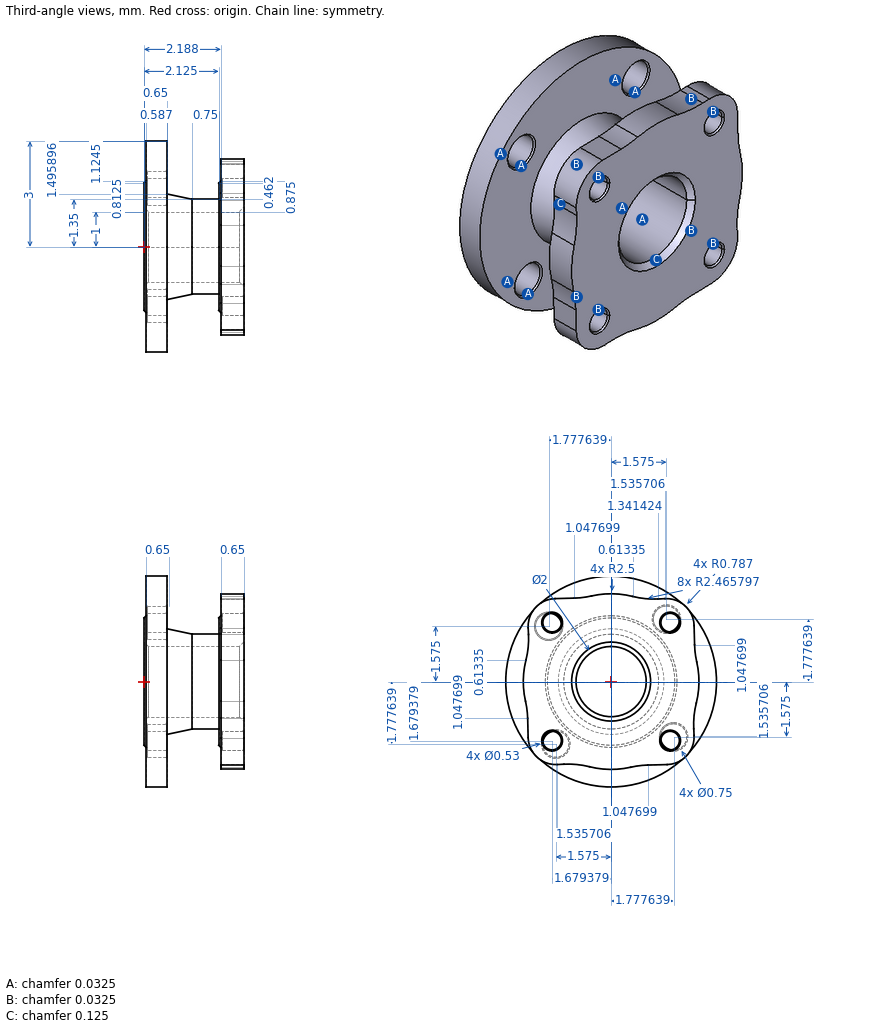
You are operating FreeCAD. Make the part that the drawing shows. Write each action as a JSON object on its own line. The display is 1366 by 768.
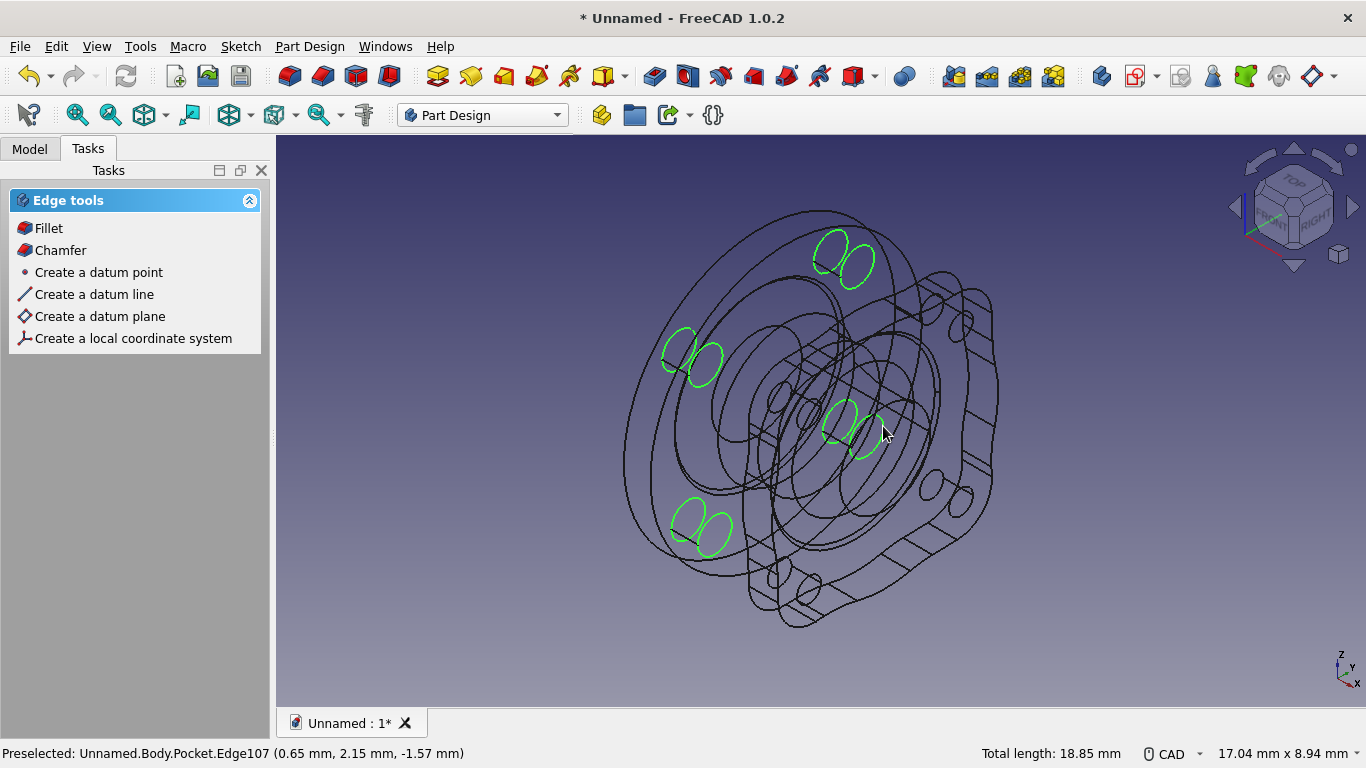
{"action": "key", "text": "v 1"}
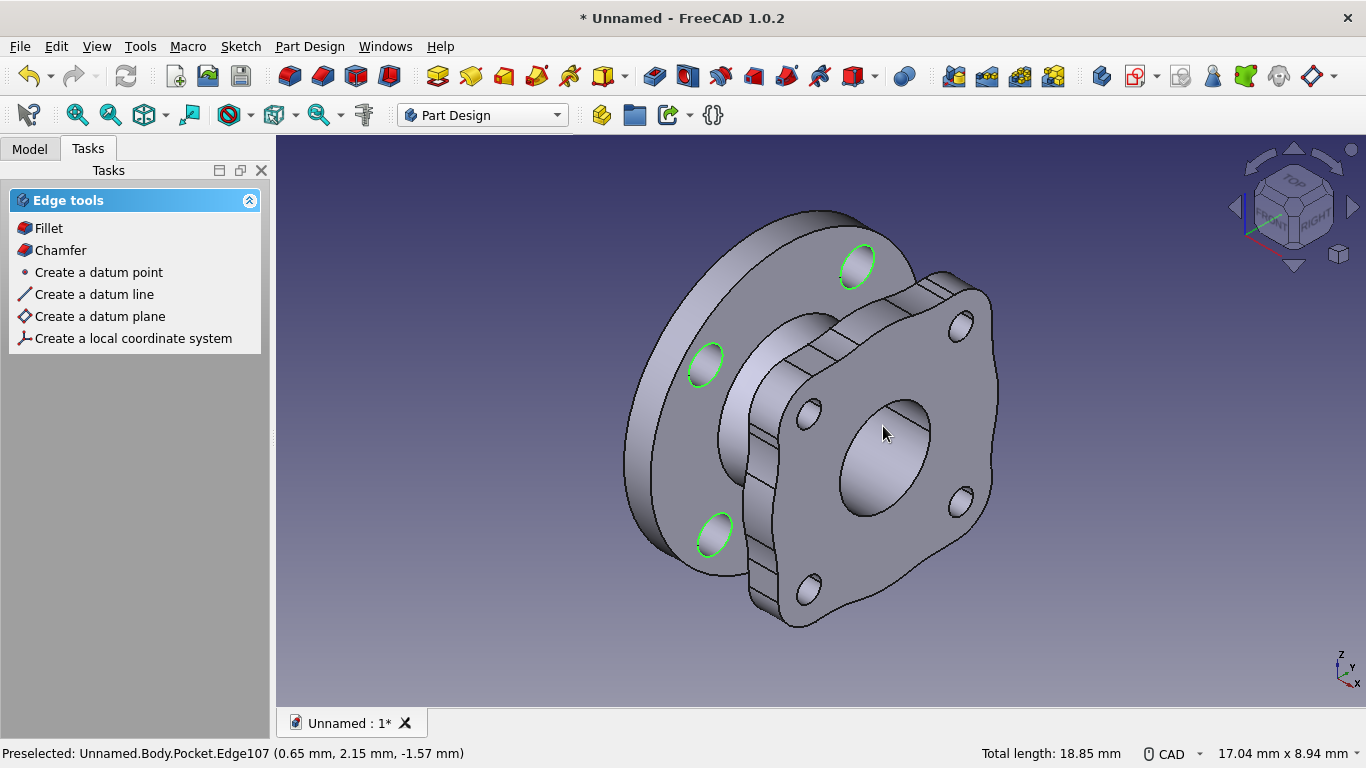
{"action": "left_click", "coordinate": [323, 76]}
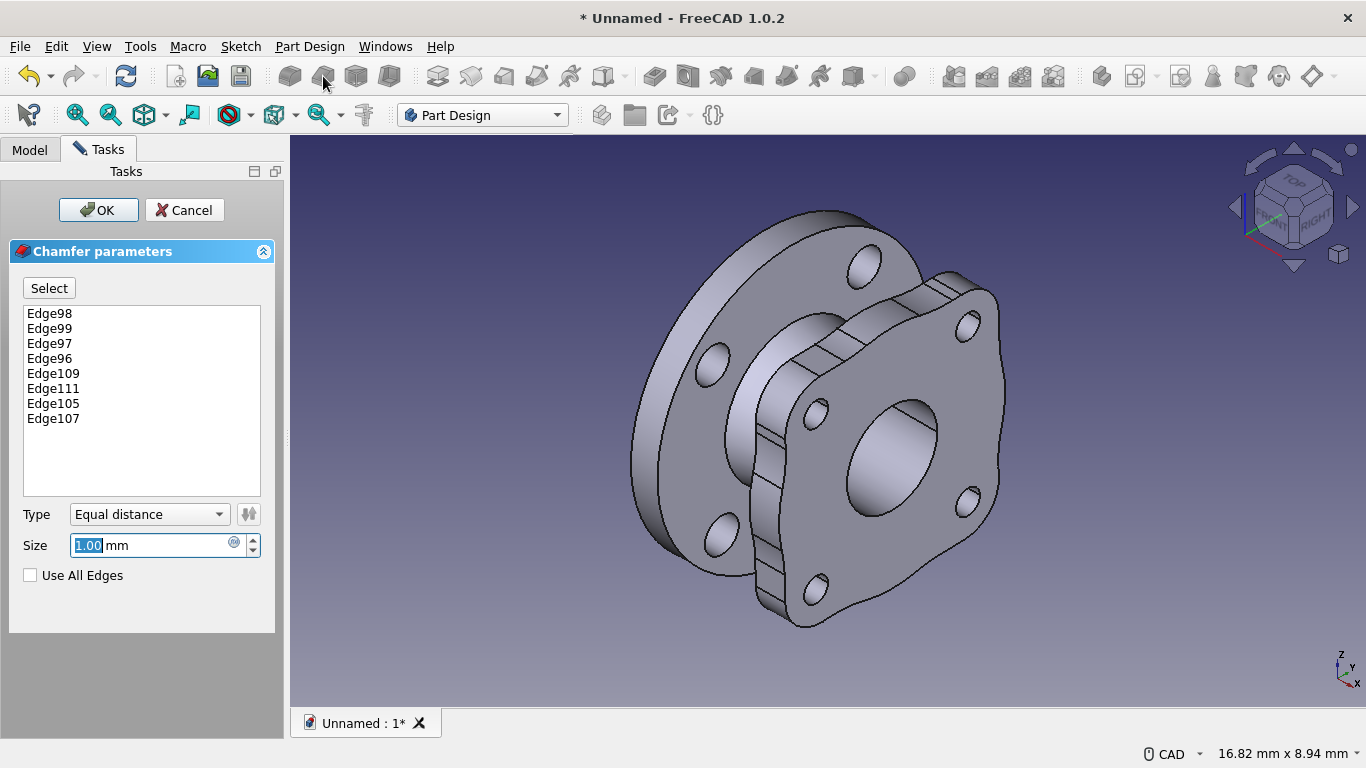
{"action": "type", "text": "0.0325"}
{"action": "key", "text": "Tab"}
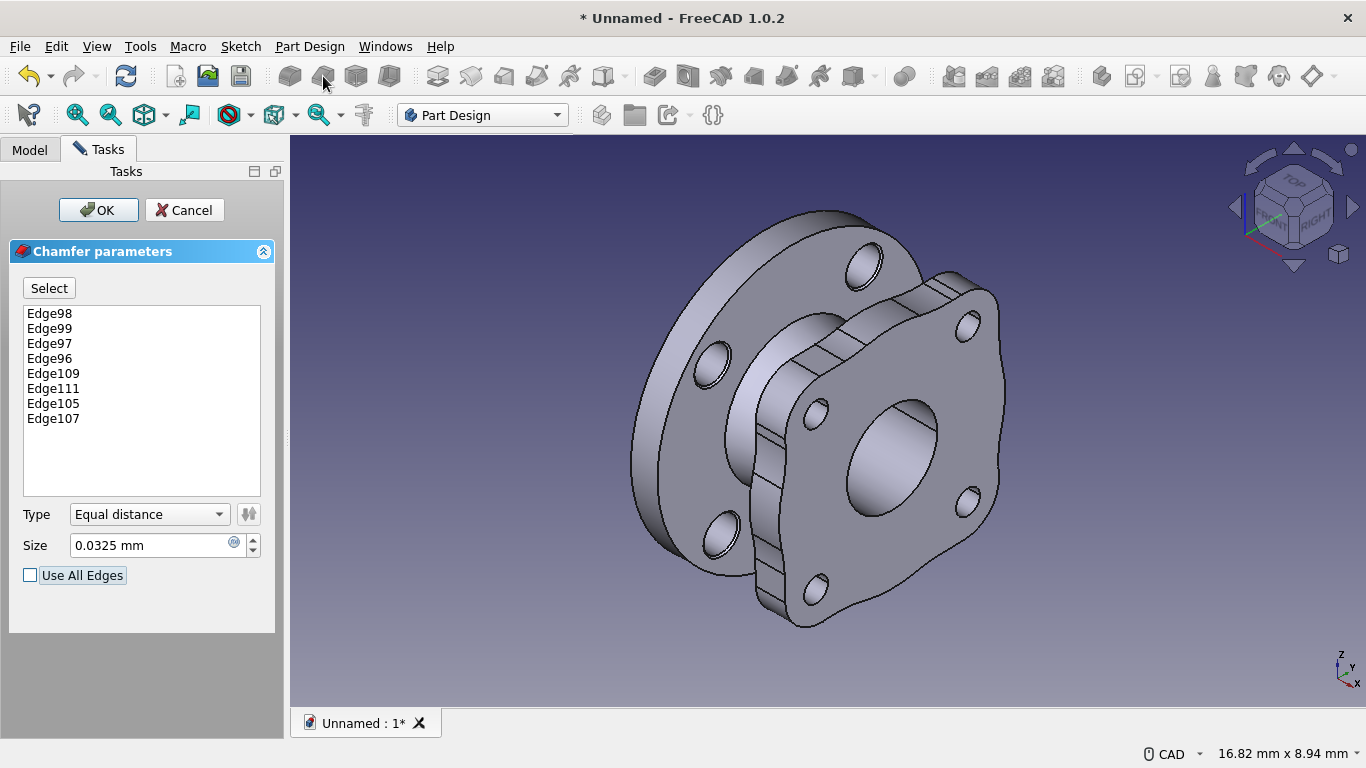
{"action": "left_click", "coordinate": [99, 210]}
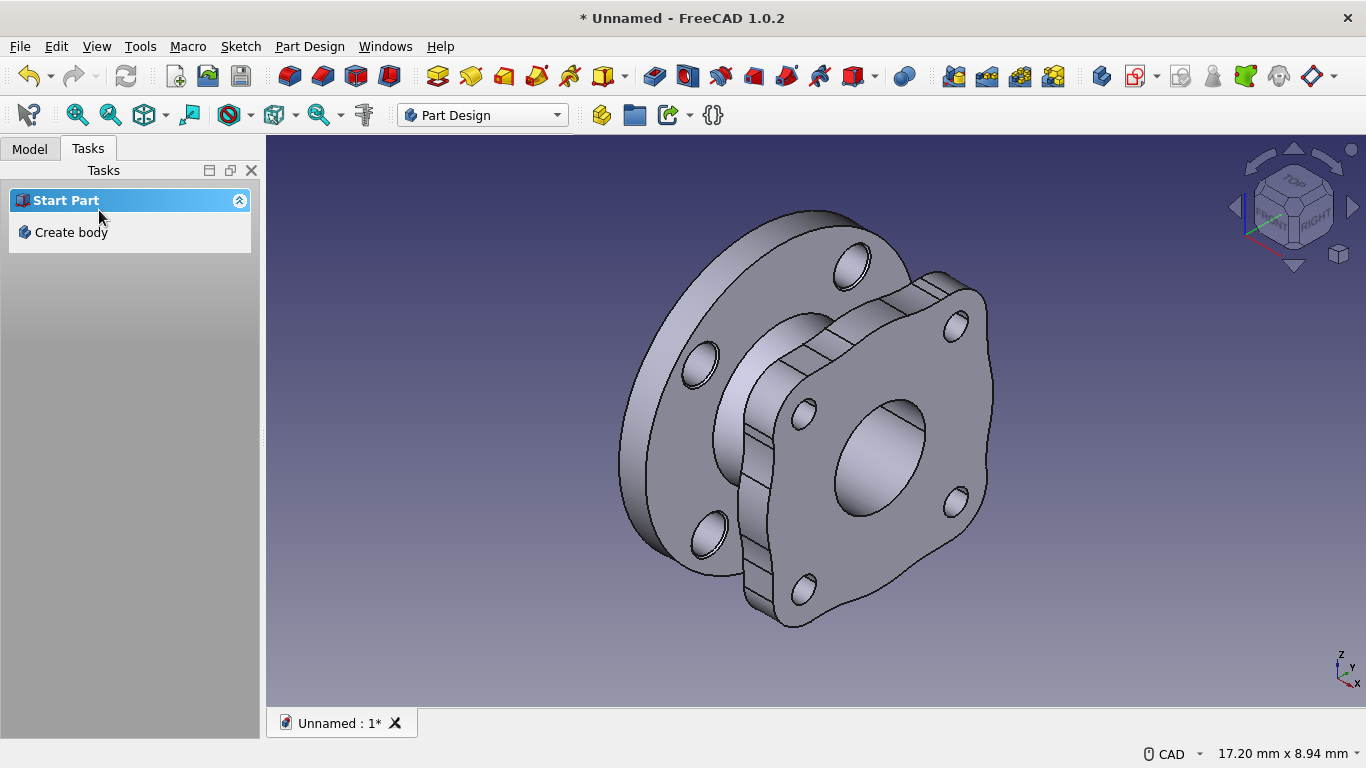
{"action": "left_click", "coordinate": [946, 339]}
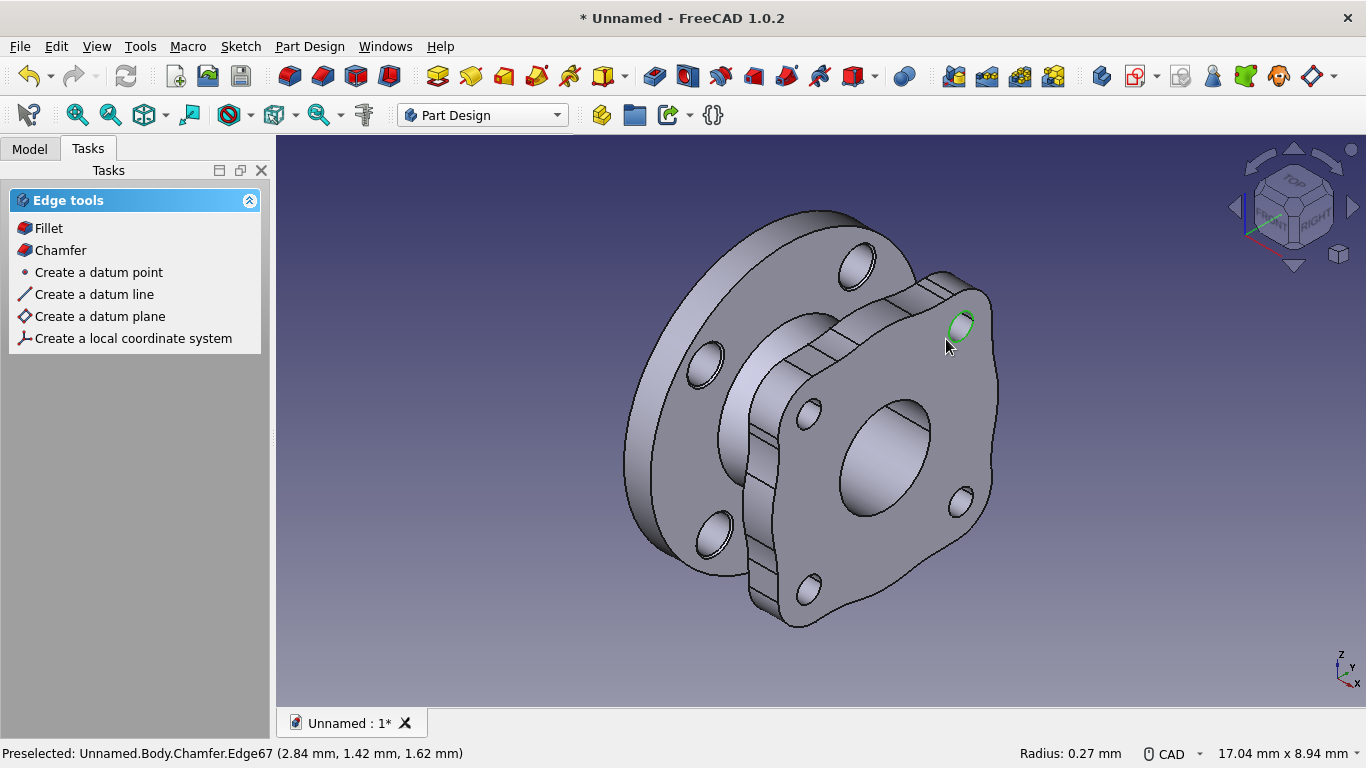
{"action": "left_click", "coordinate": [951, 515], "text": "ctrl"}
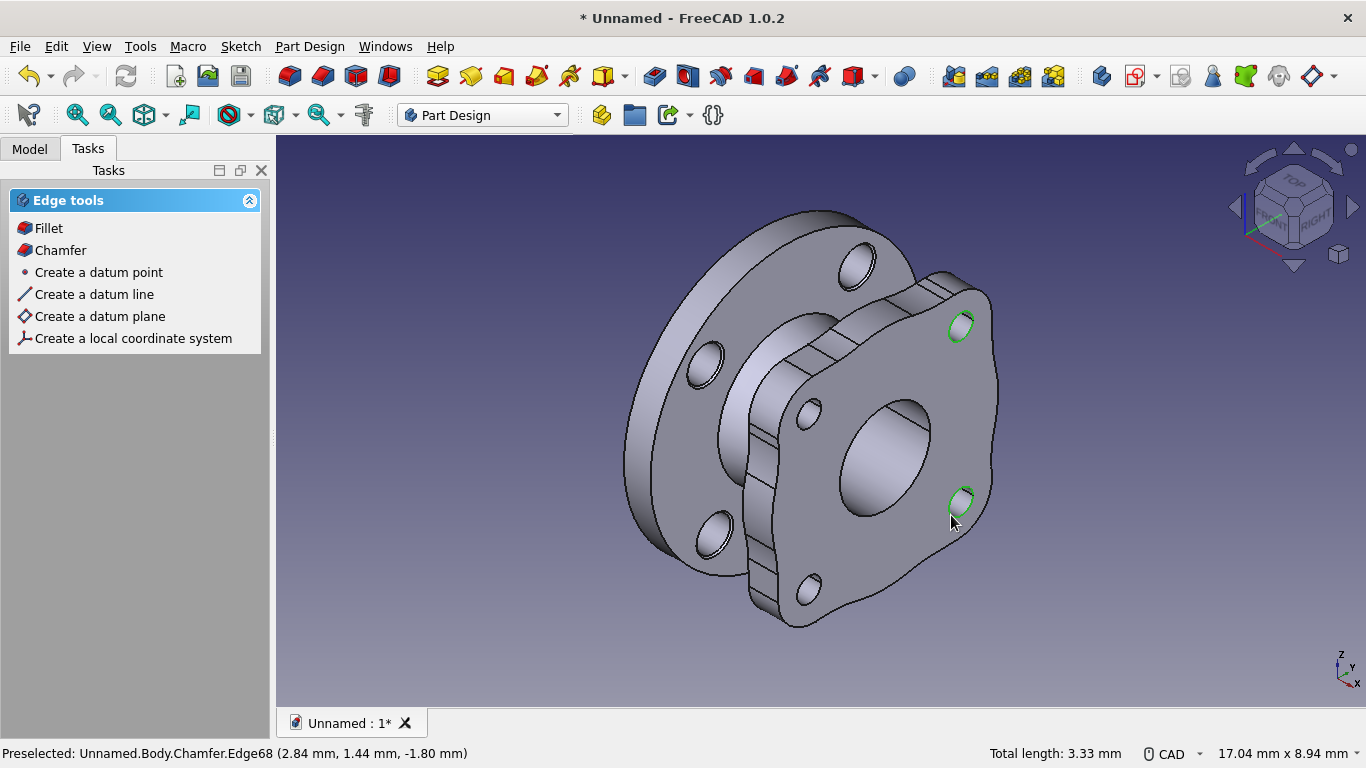
{"action": "left_click", "coordinate": [799, 602], "text": "ctrl"}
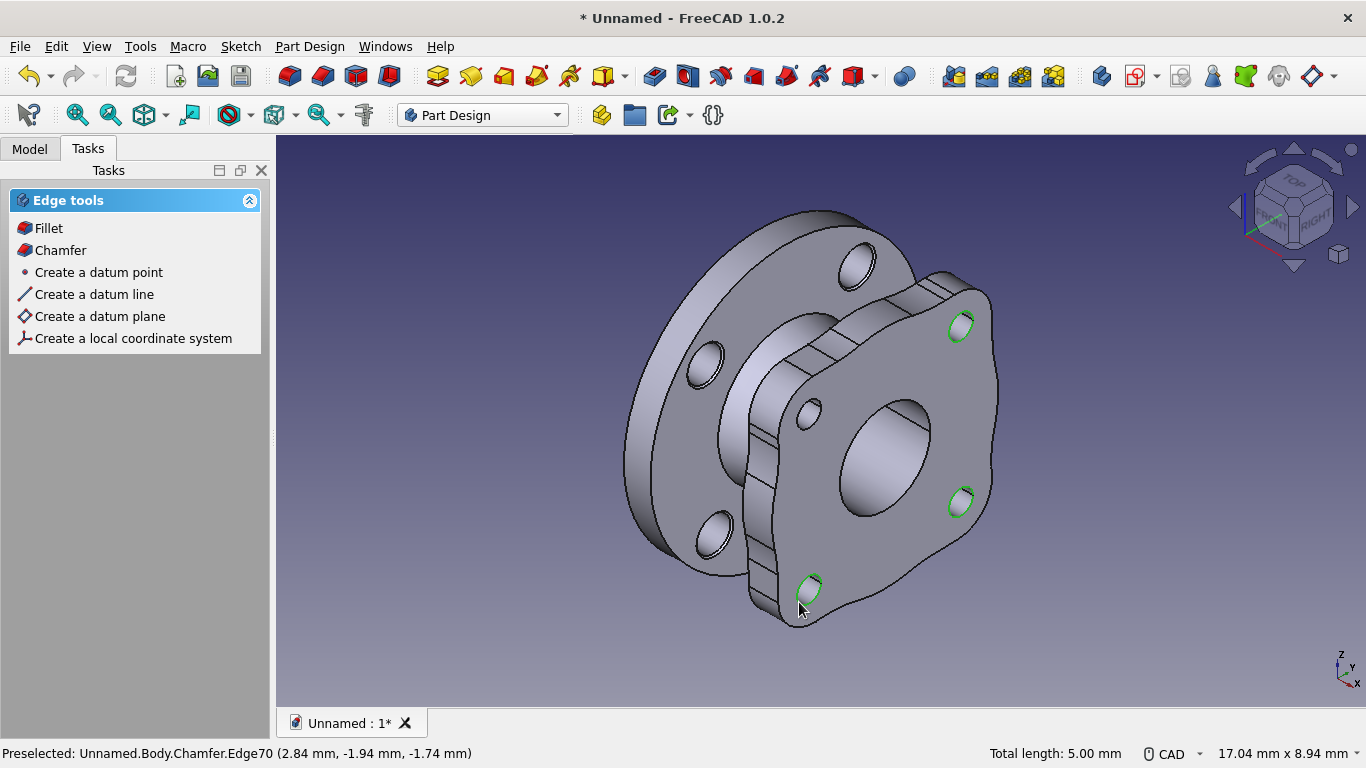
{"action": "left_click", "coordinate": [799, 427], "text": "ctrl"}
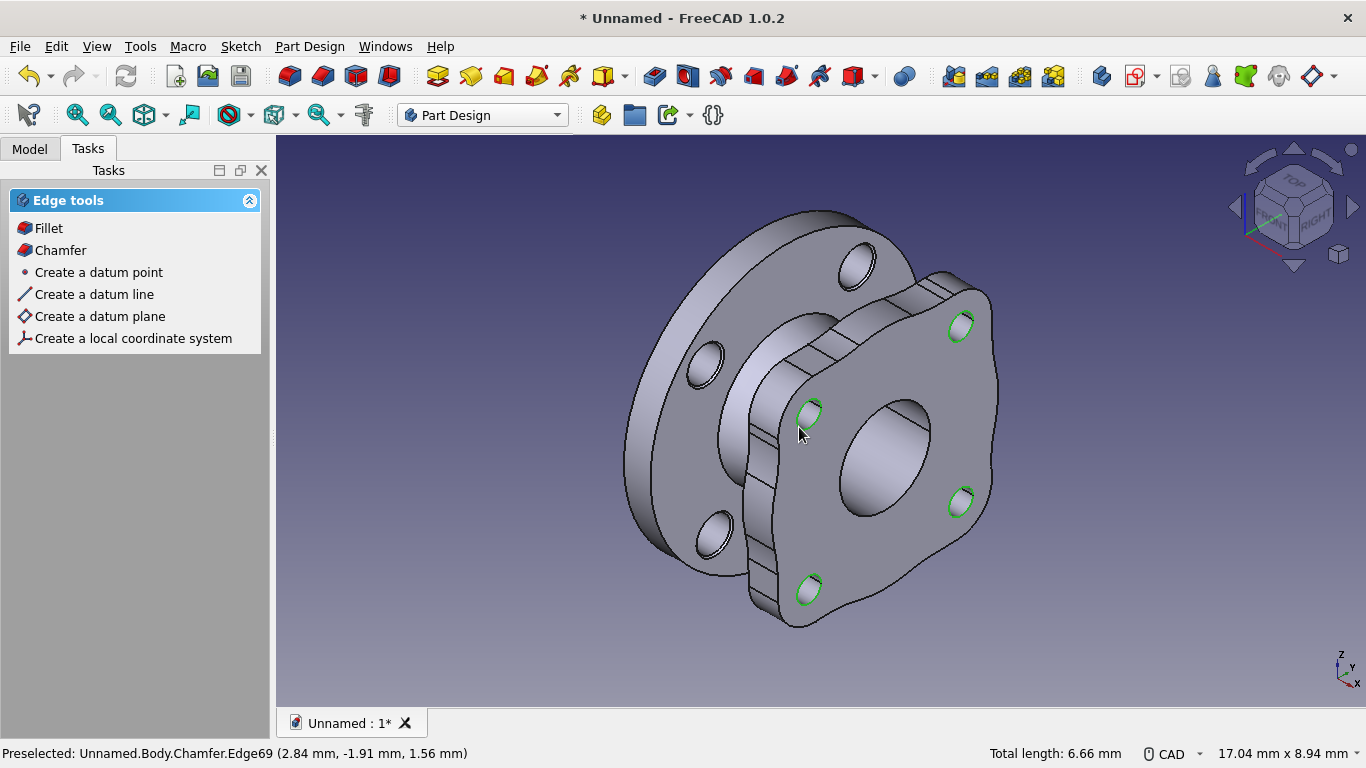
{"action": "key", "text": "2"}